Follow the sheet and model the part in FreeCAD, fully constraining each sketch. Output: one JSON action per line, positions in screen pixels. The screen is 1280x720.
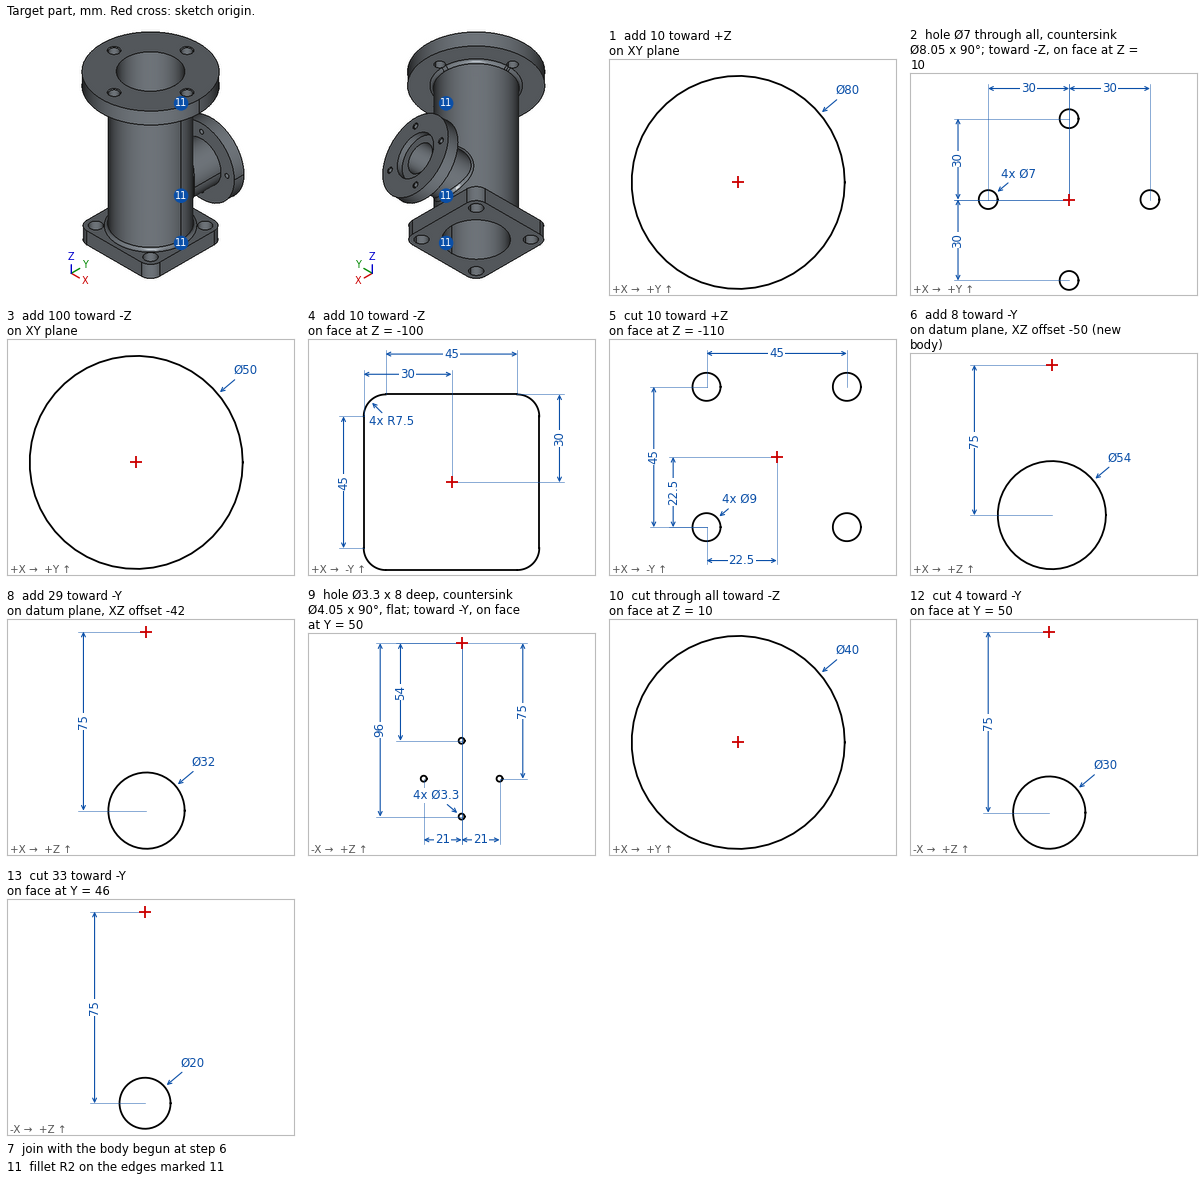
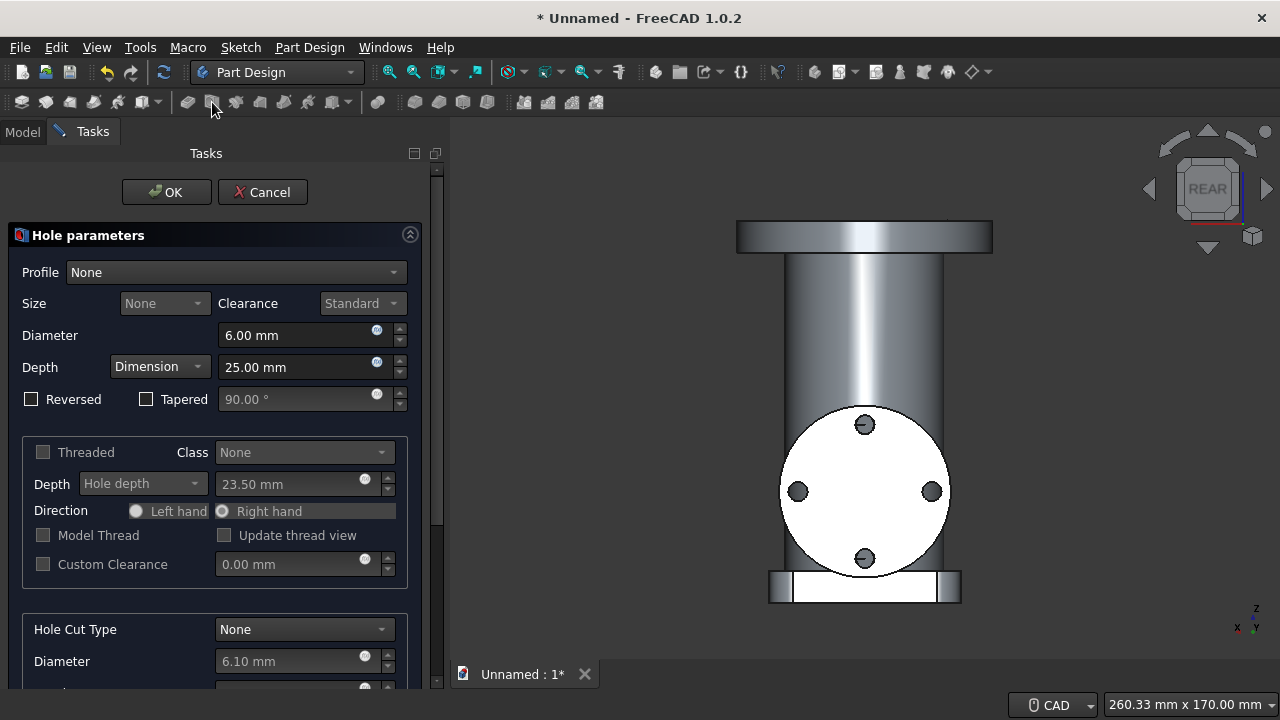
{"action": "triple_click", "coordinate": [305, 335]}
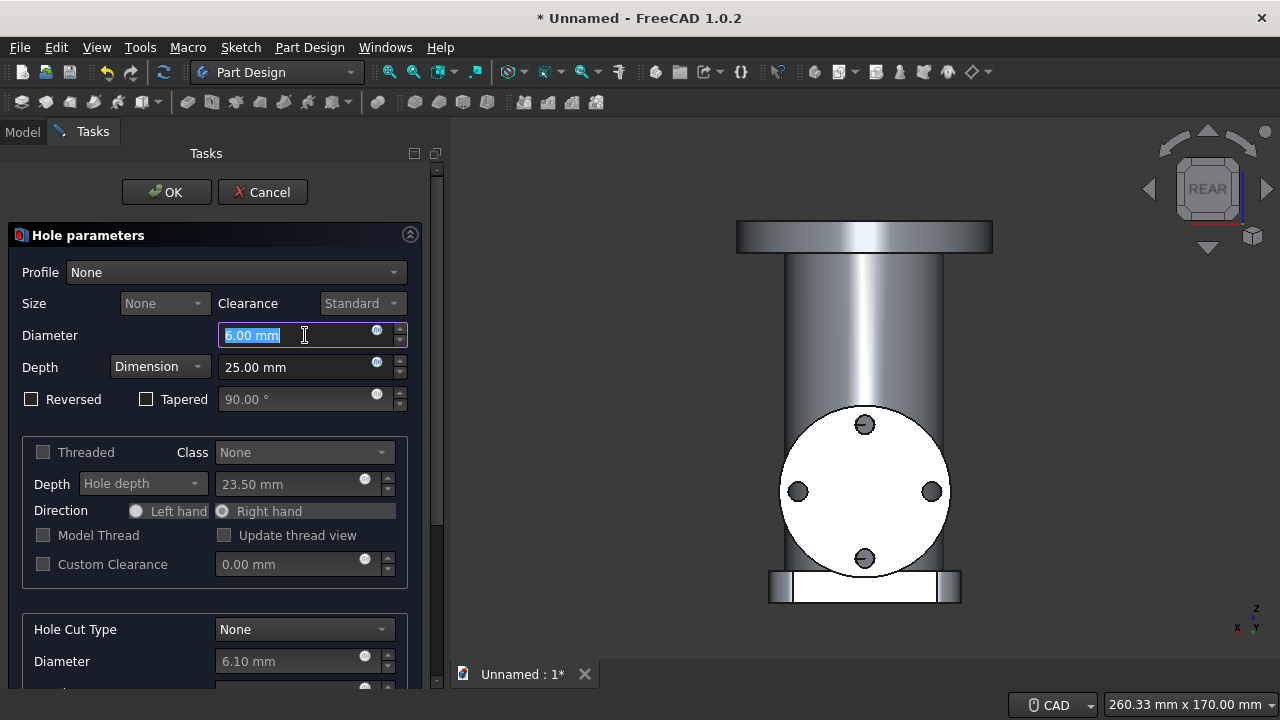
{"action": "type", "text": "3.3"}
{"action": "key", "text": "Tab"}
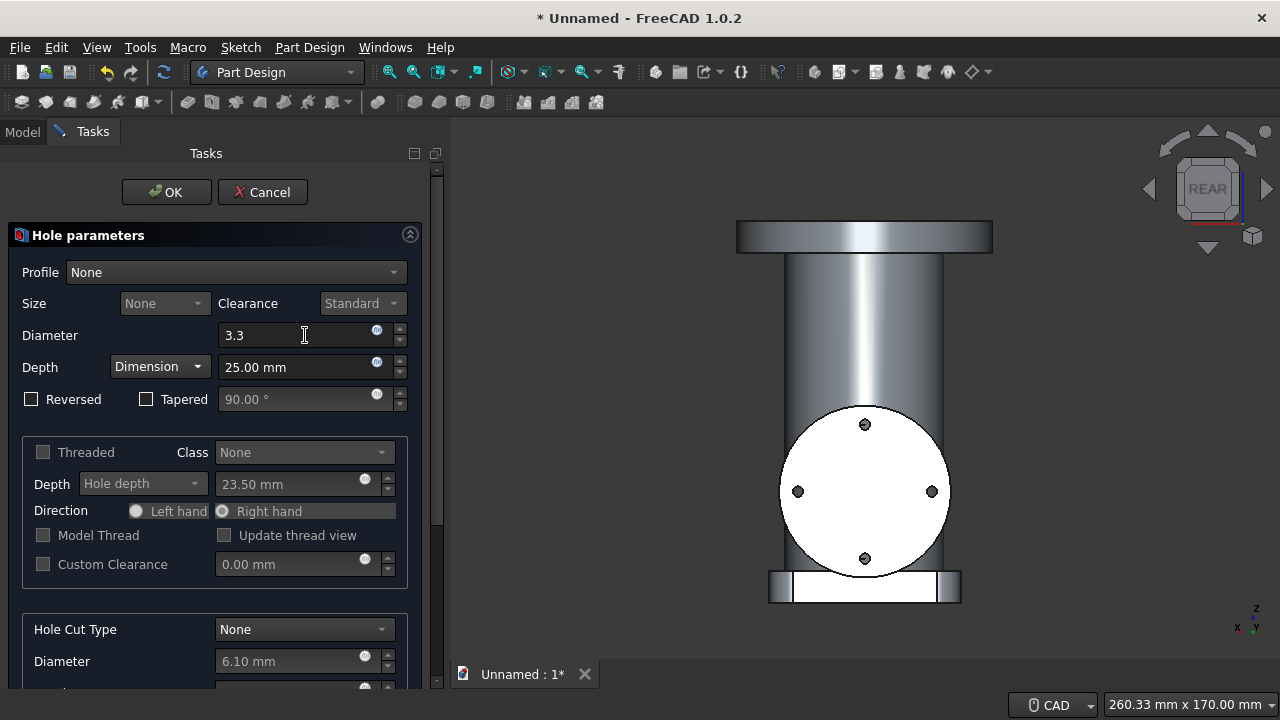
{"action": "triple_click", "coordinate": [305, 367]}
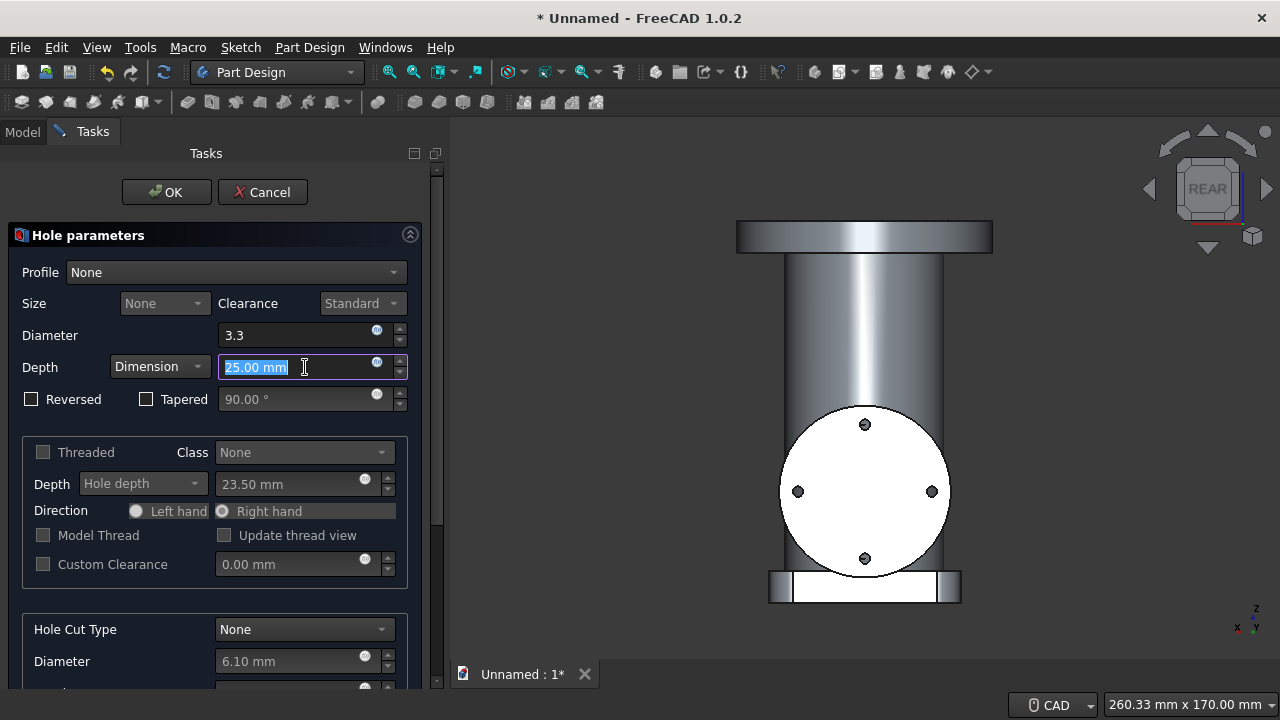
{"action": "type", "text": "8"}
{"action": "key", "text": "Tab"}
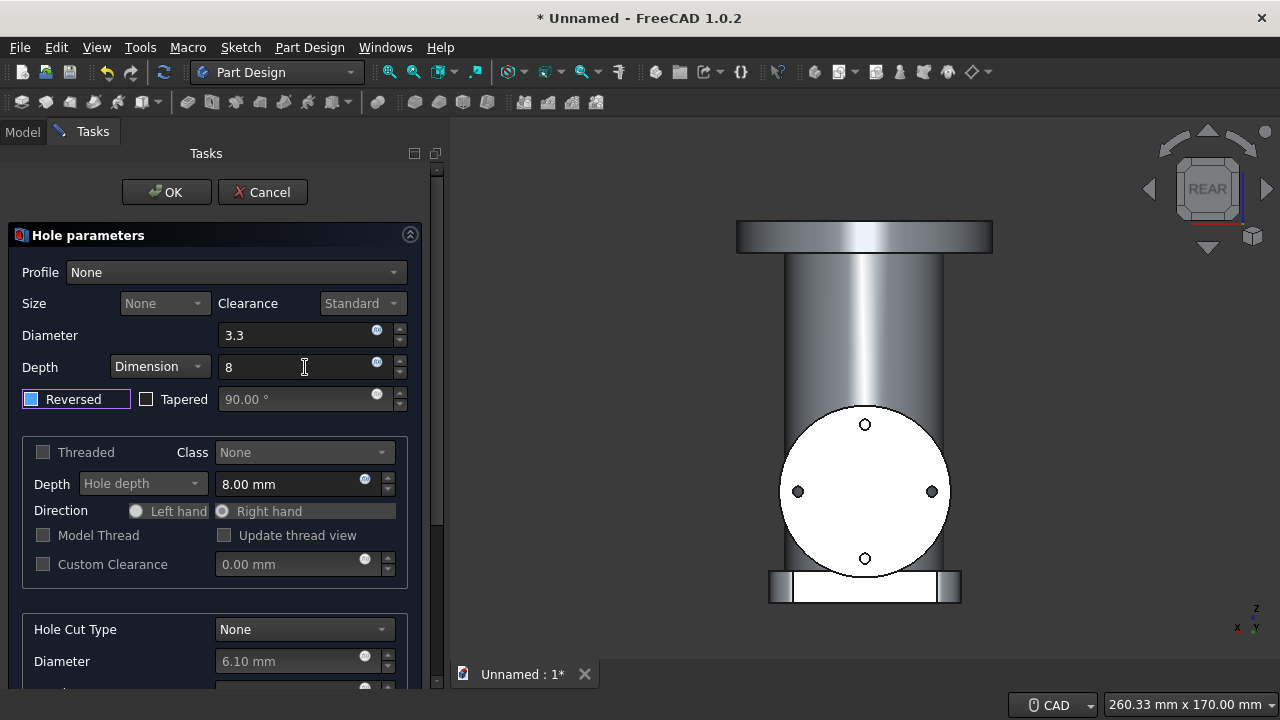
{"action": "left_click", "coordinate": [306, 630]}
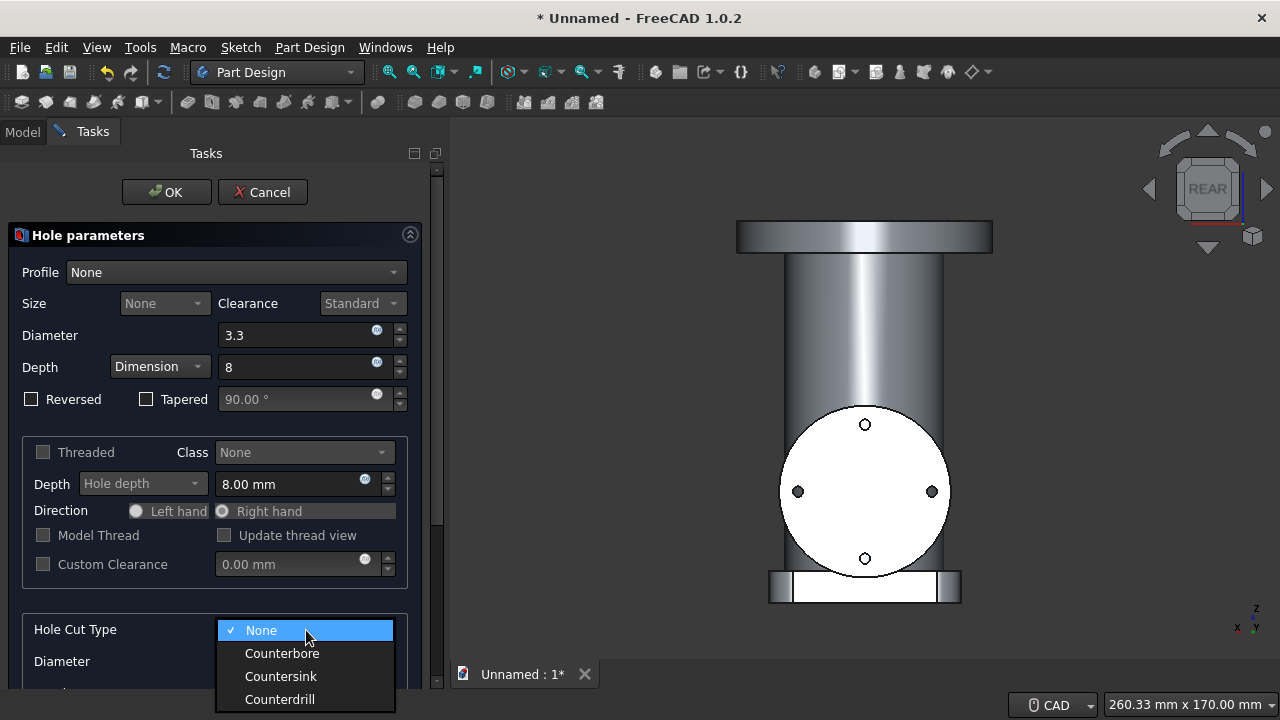
{"action": "left_click", "coordinate": [304, 676]}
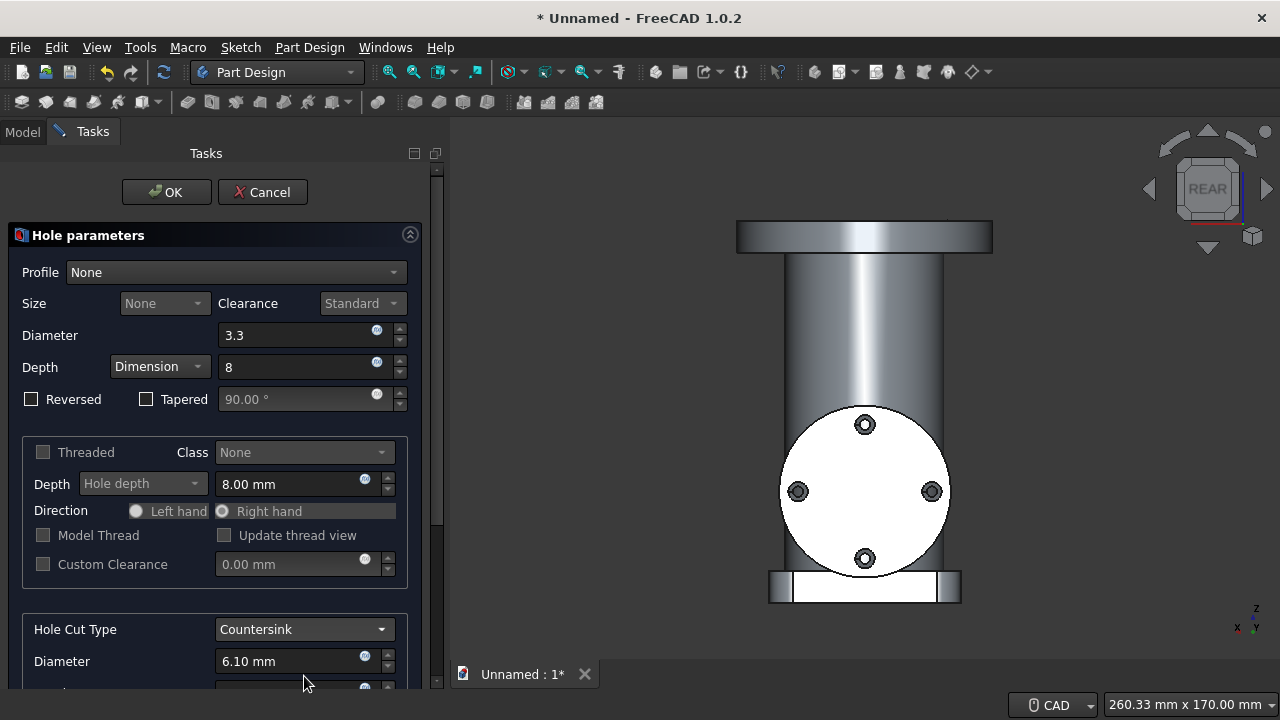
{"action": "triple_click", "coordinate": [298, 661]}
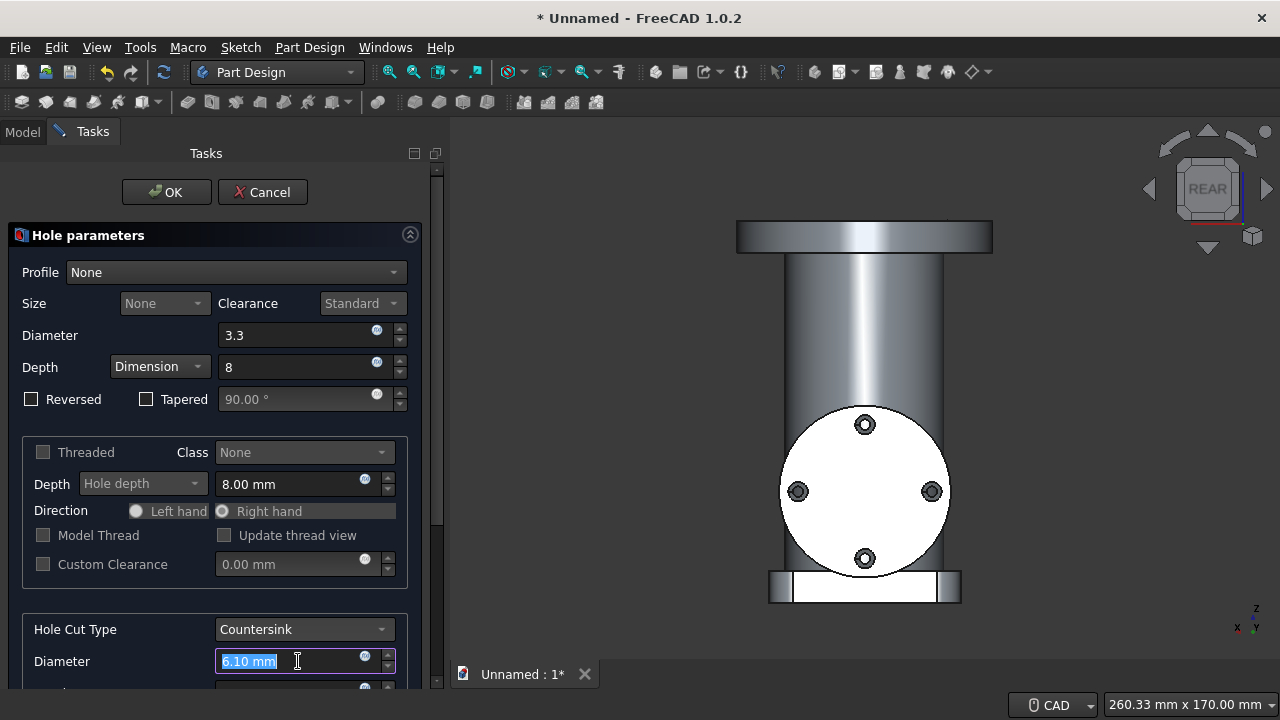
{"action": "type", "text": "4.05"}
{"action": "key", "text": "Tab"}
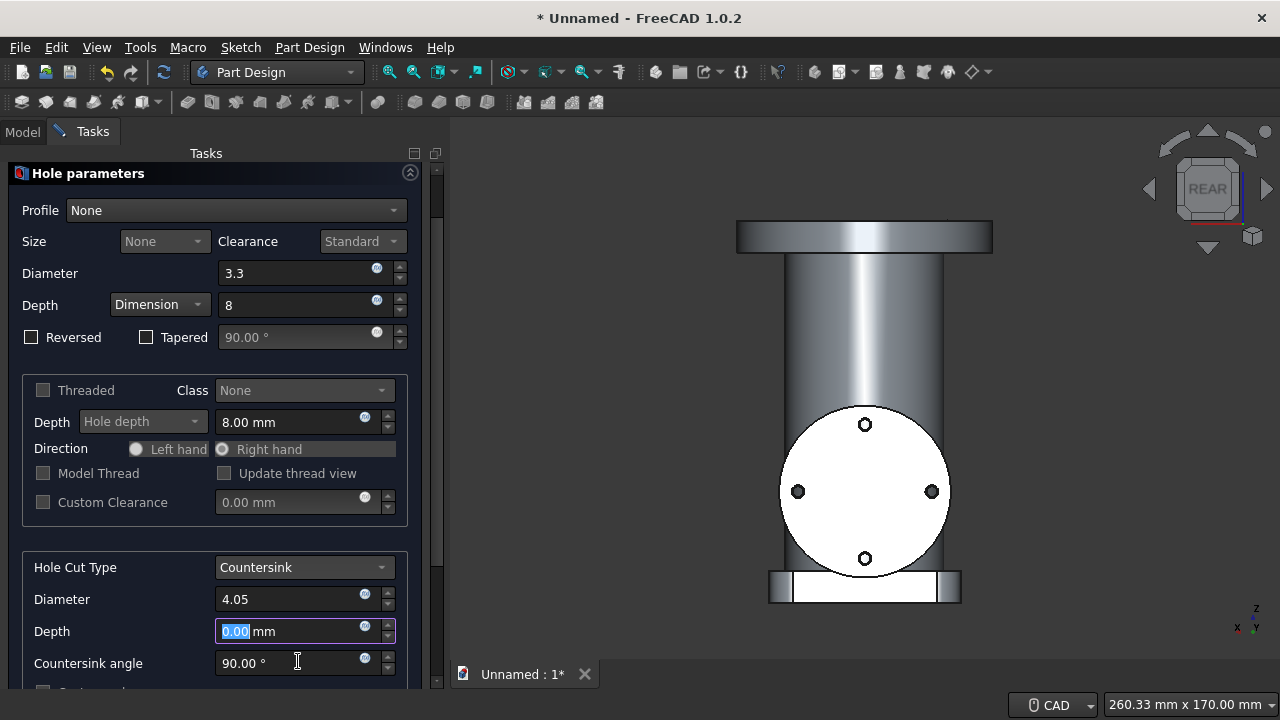
{"action": "scroll", "coordinate": [437, 426], "scroll_direction": "down", "scroll_amount": 3}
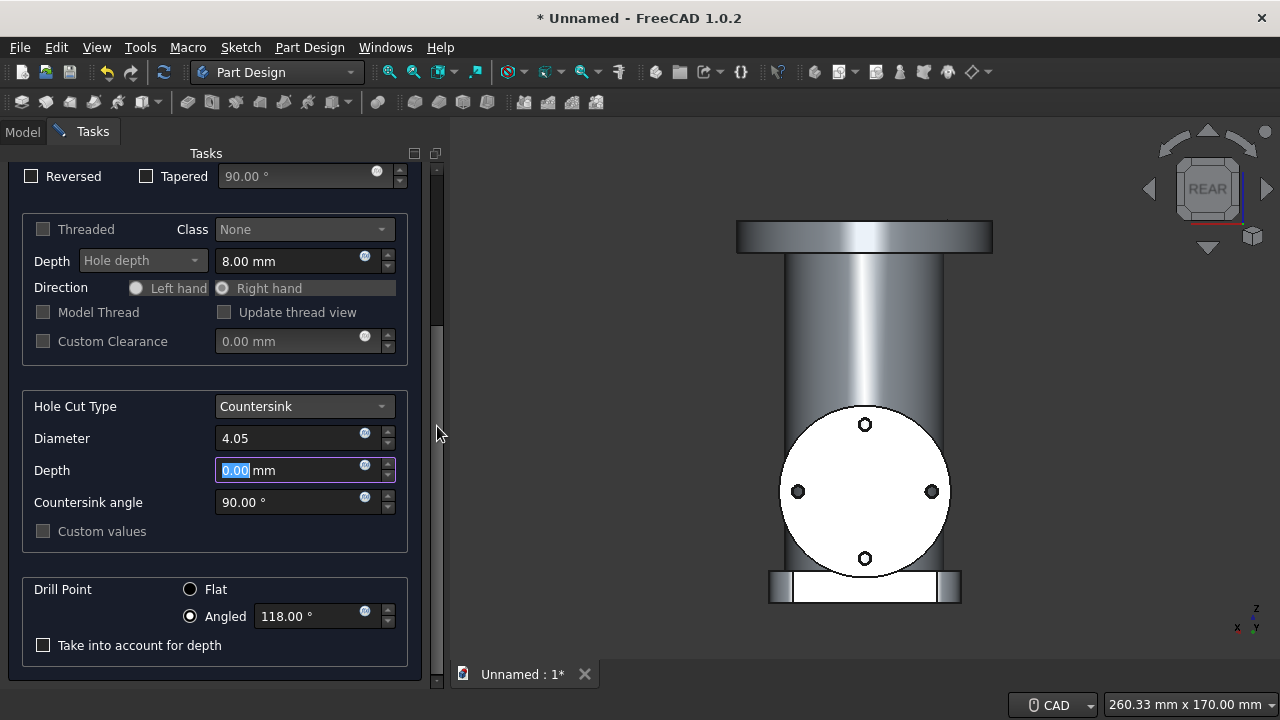
{"action": "left_click", "coordinate": [191, 589]}